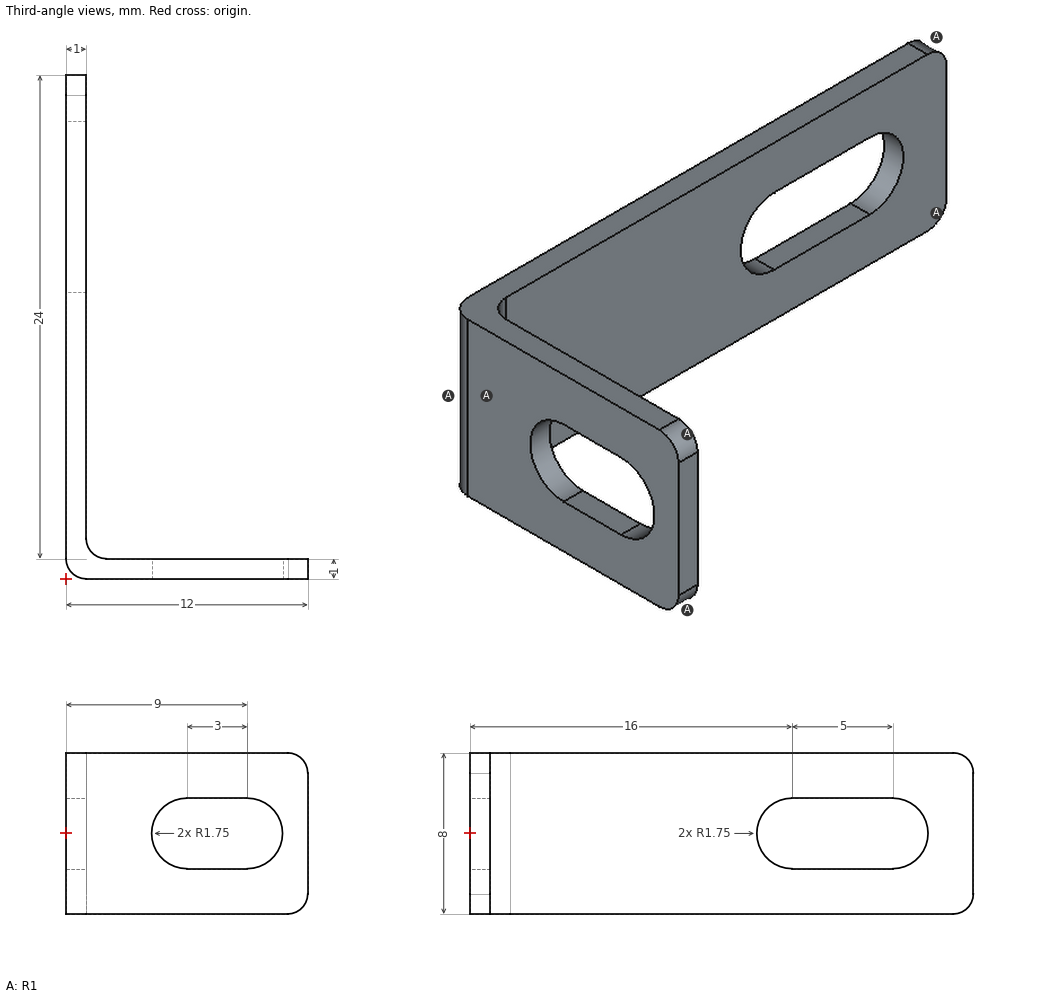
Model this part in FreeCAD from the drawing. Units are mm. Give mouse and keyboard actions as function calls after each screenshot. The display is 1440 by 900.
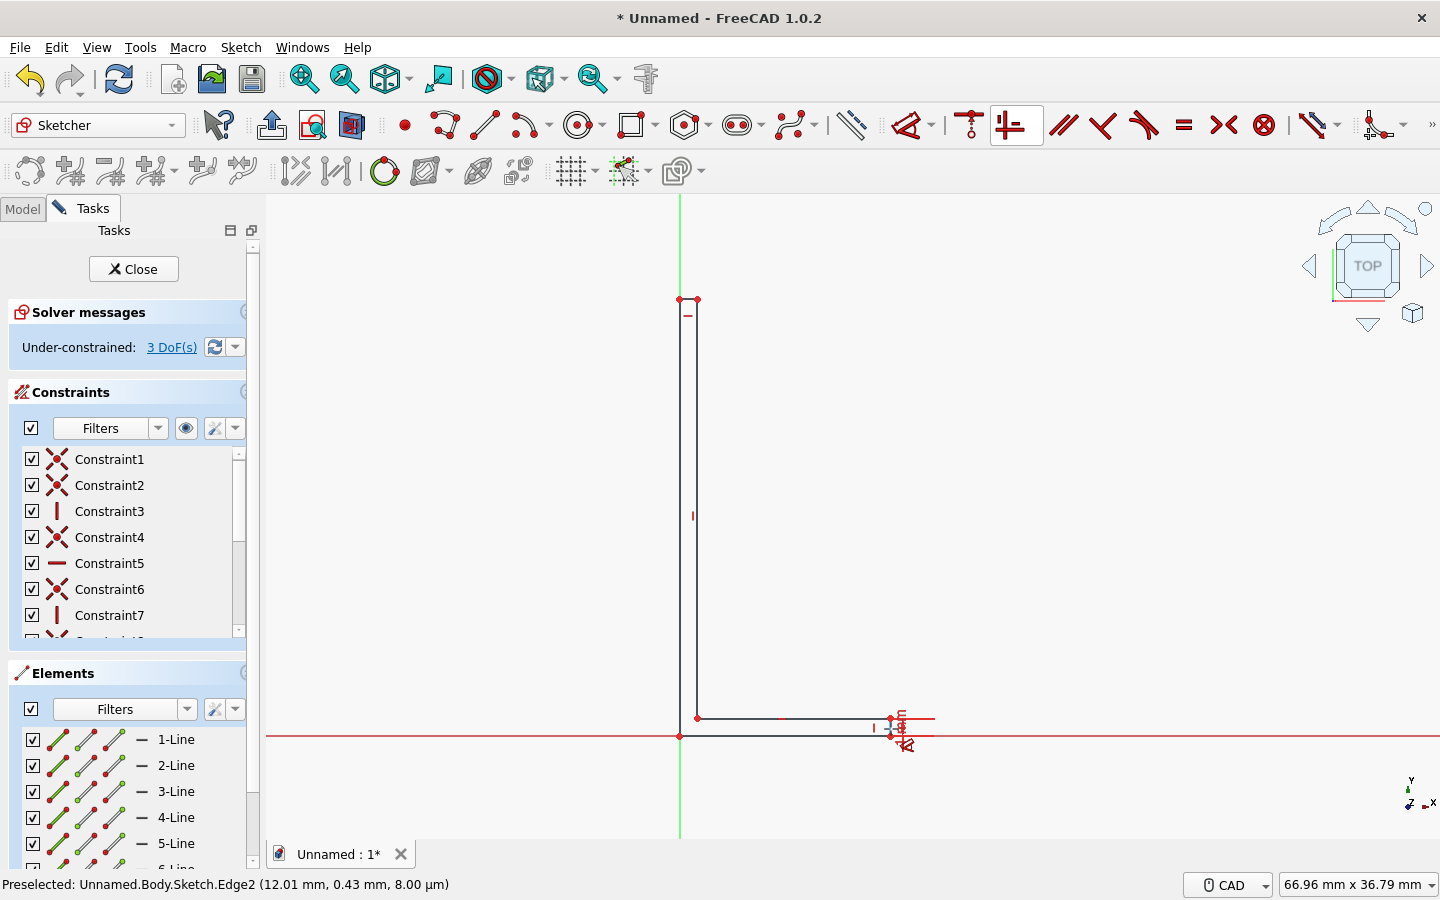
scroll(692, 299, up, 5)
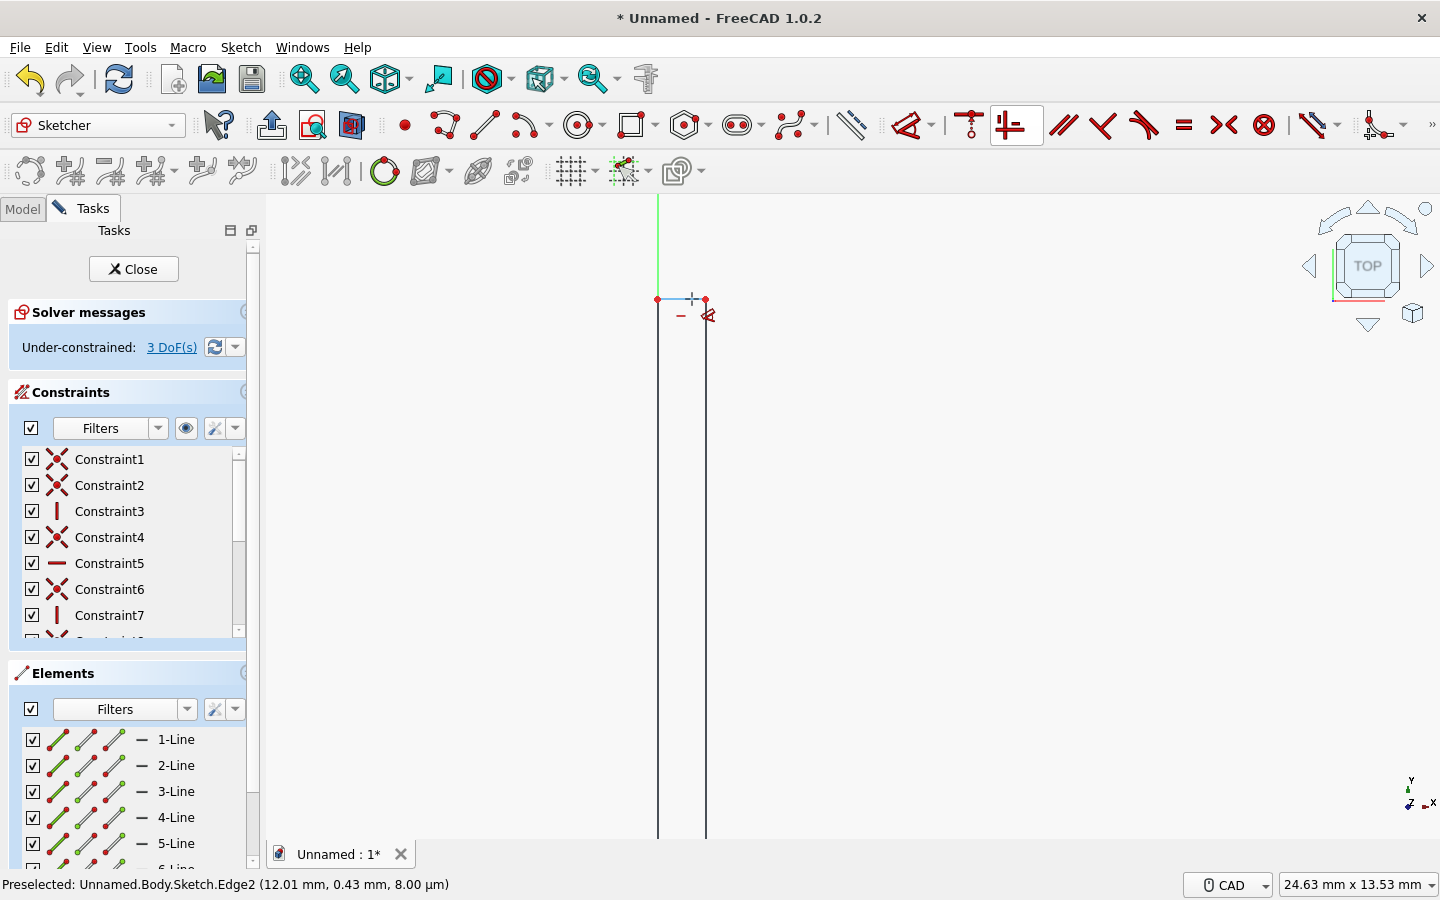
click(691, 299)
click(682, 265)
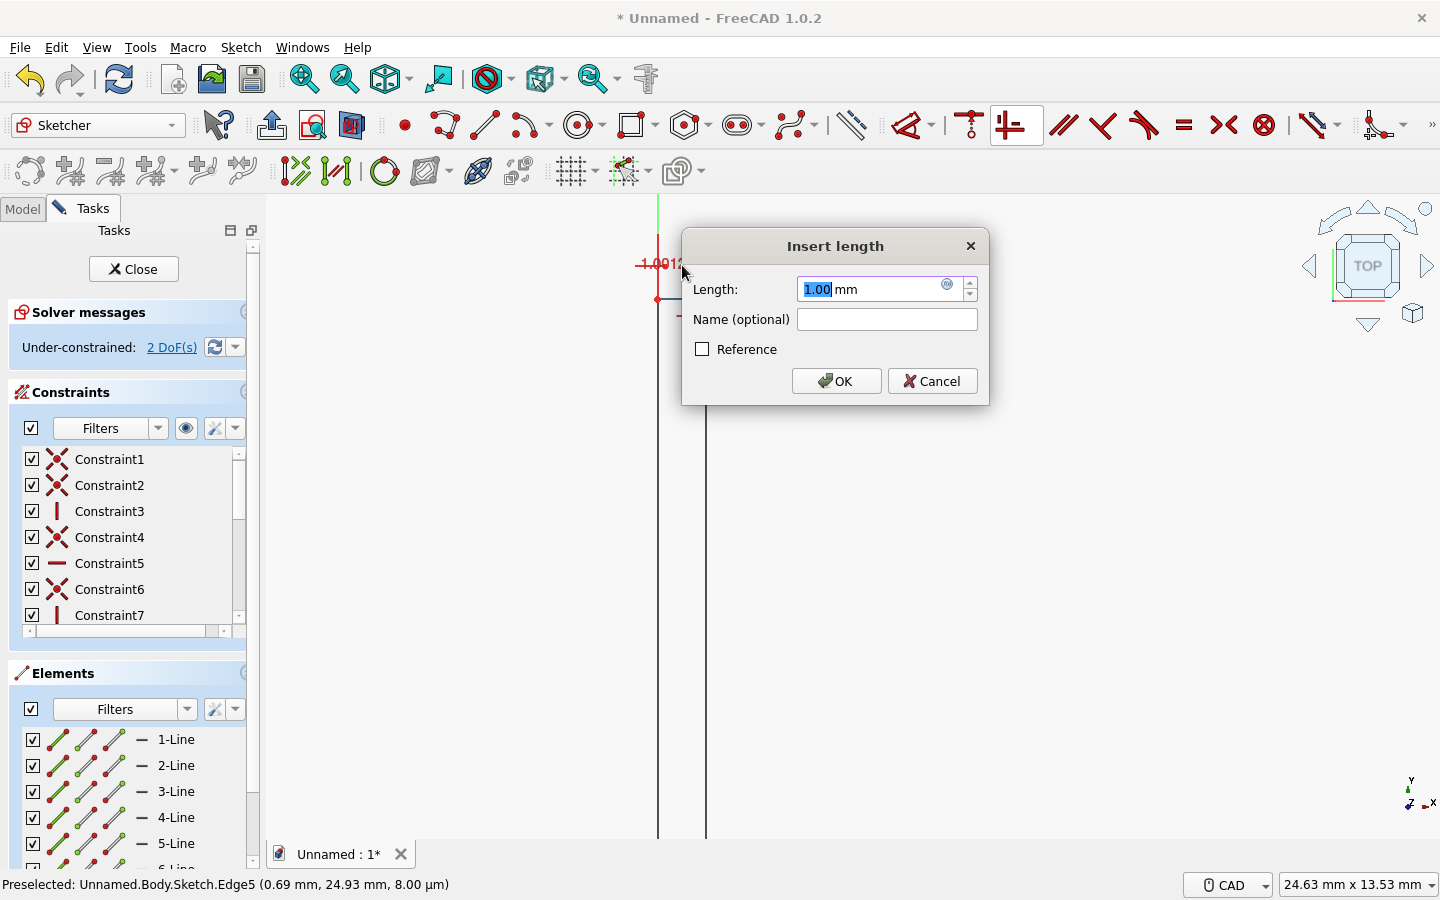
text(1)
key(Return)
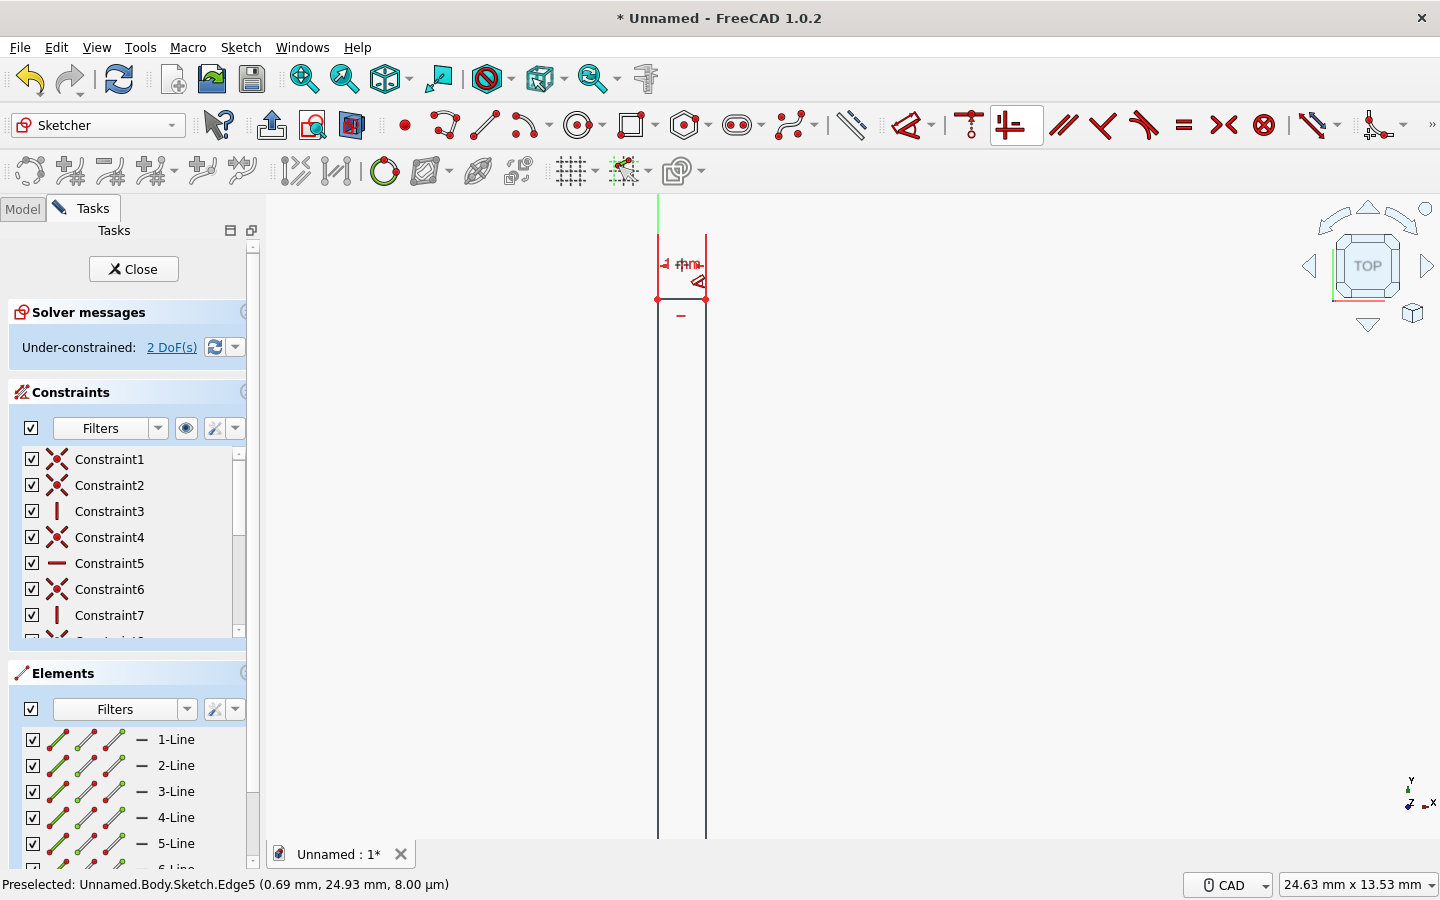
scroll(692, 298, down, 5)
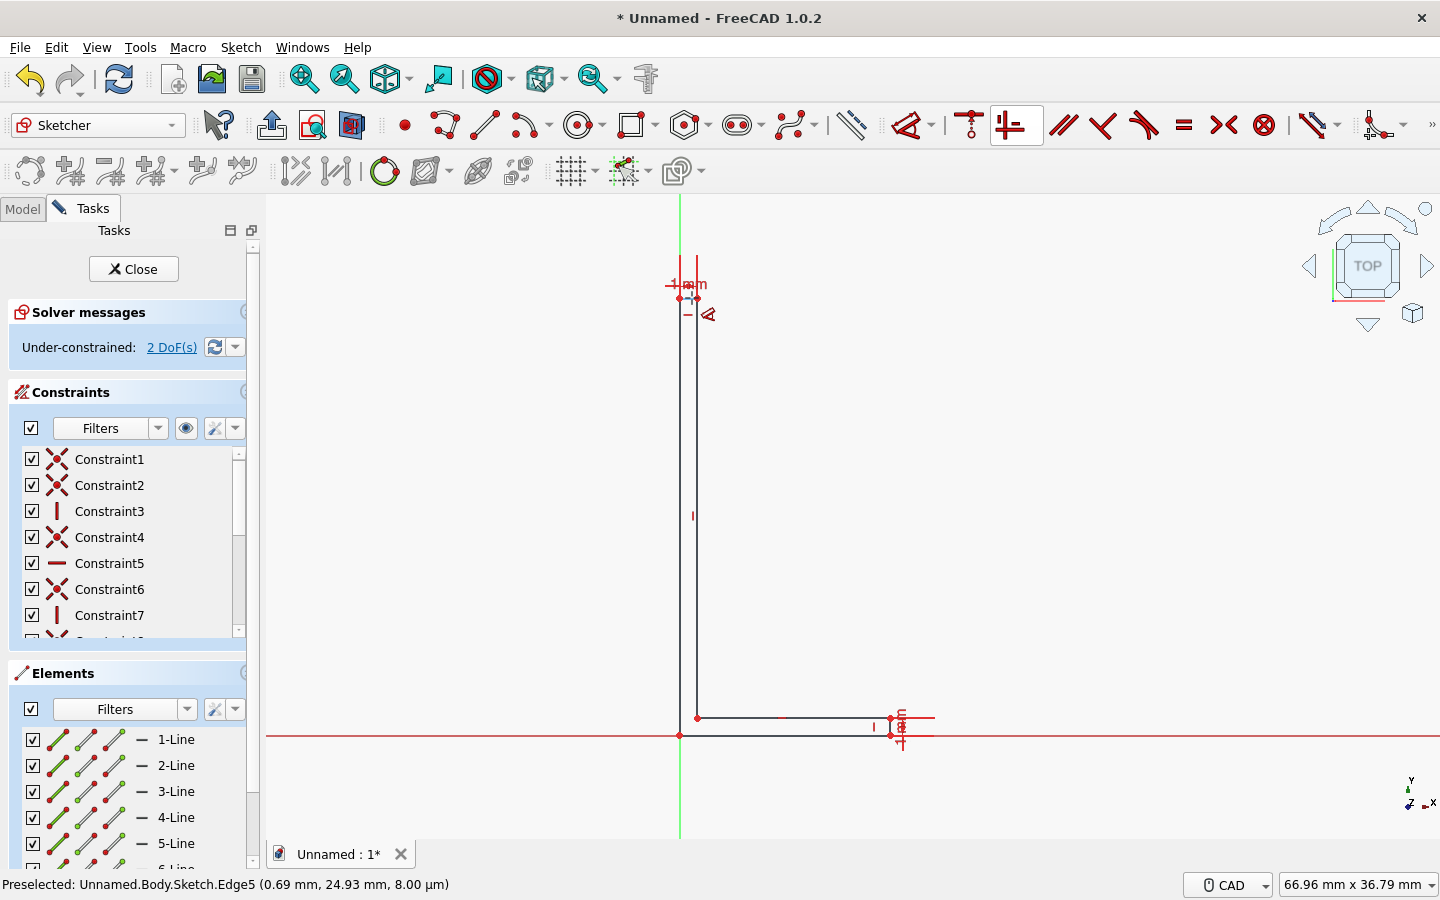
click(743, 736)
click(785, 770)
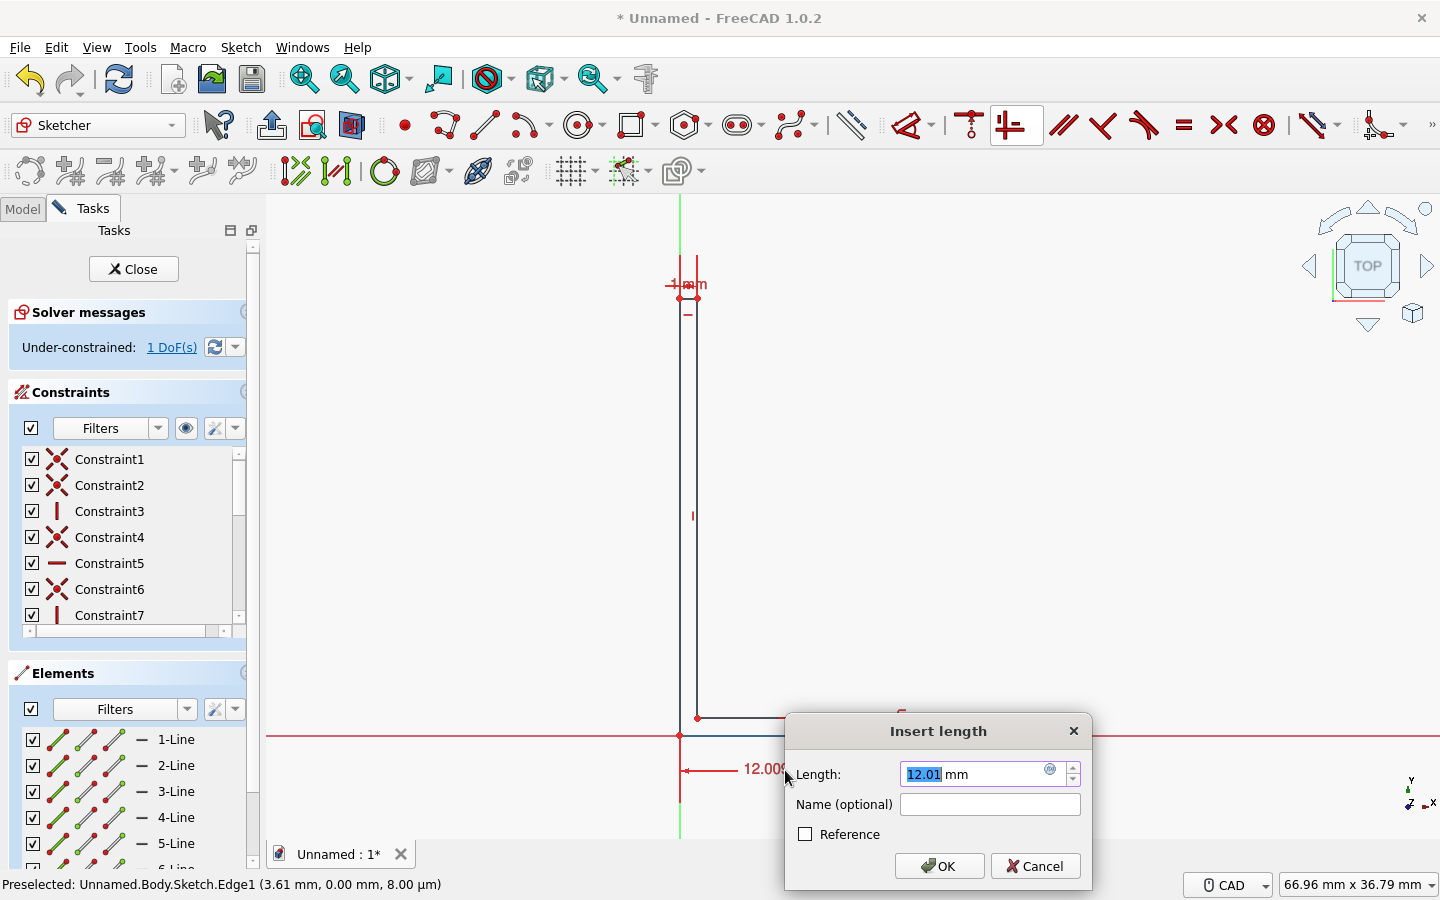
text(12)
key(Return)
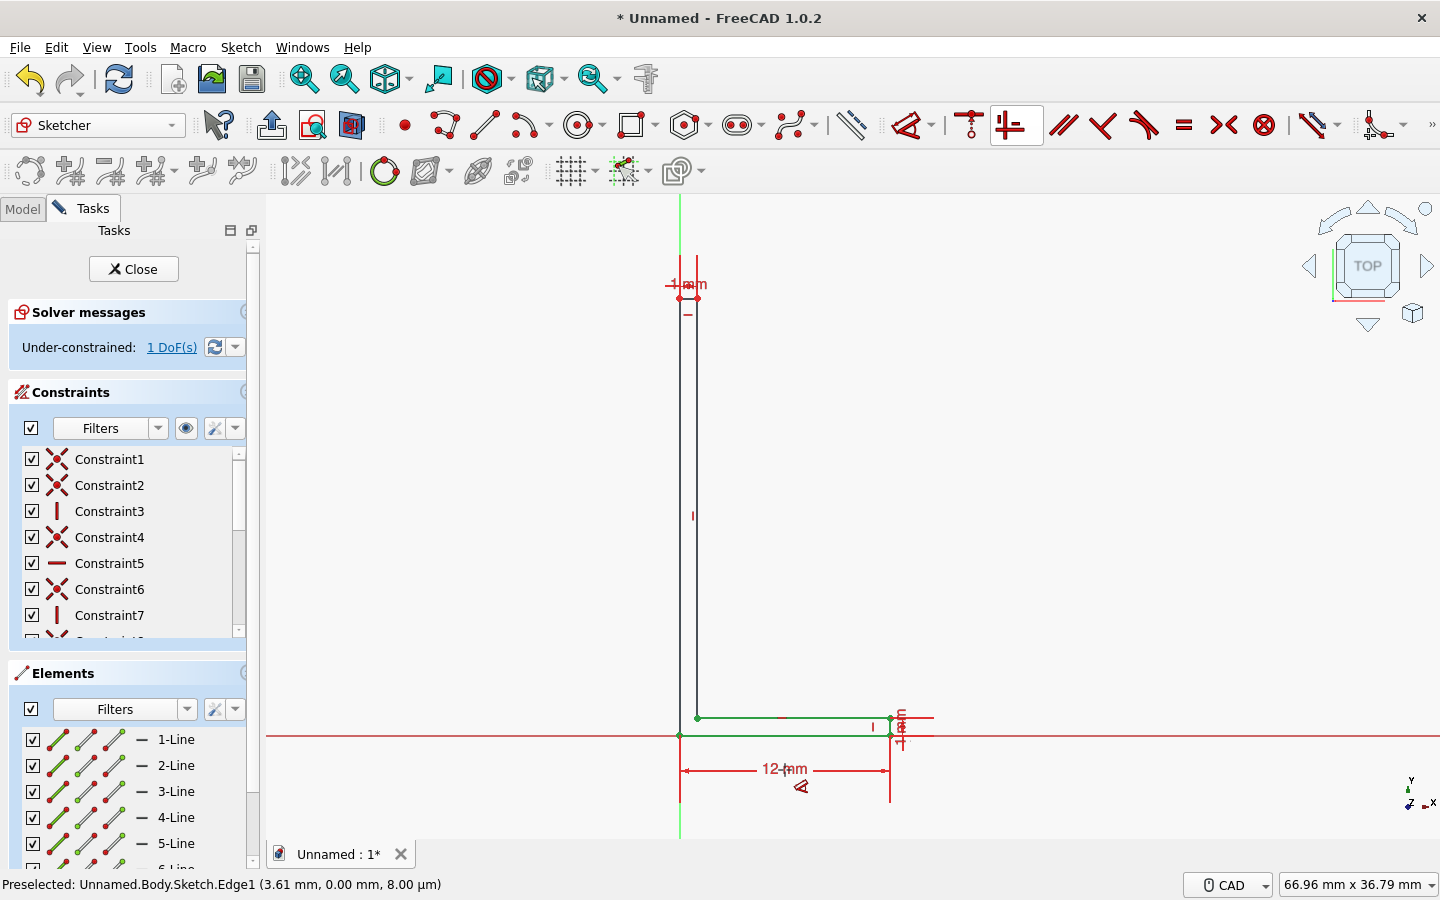
click(697, 592)
click(663, 508)